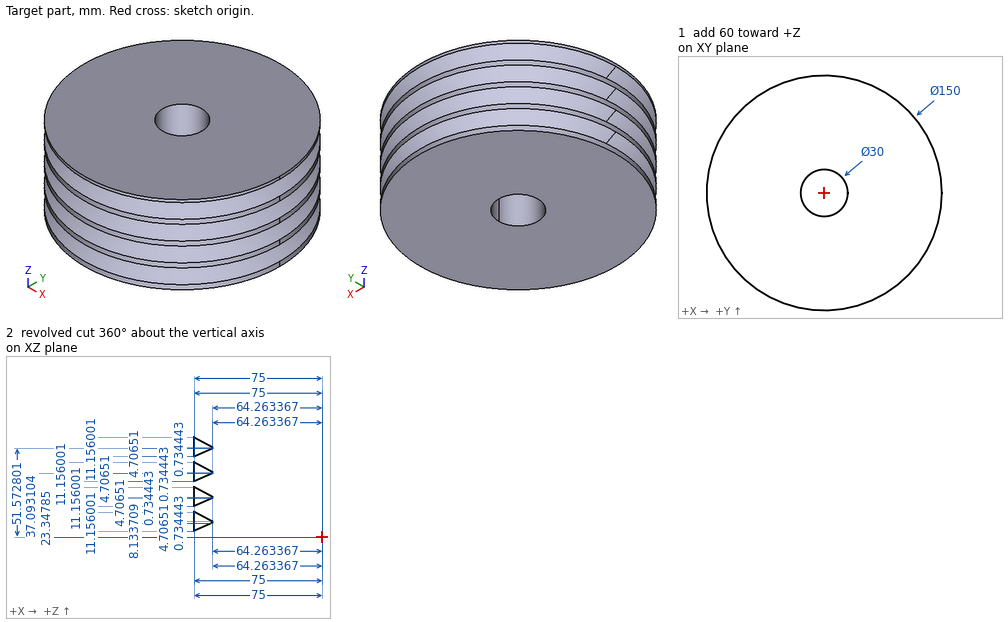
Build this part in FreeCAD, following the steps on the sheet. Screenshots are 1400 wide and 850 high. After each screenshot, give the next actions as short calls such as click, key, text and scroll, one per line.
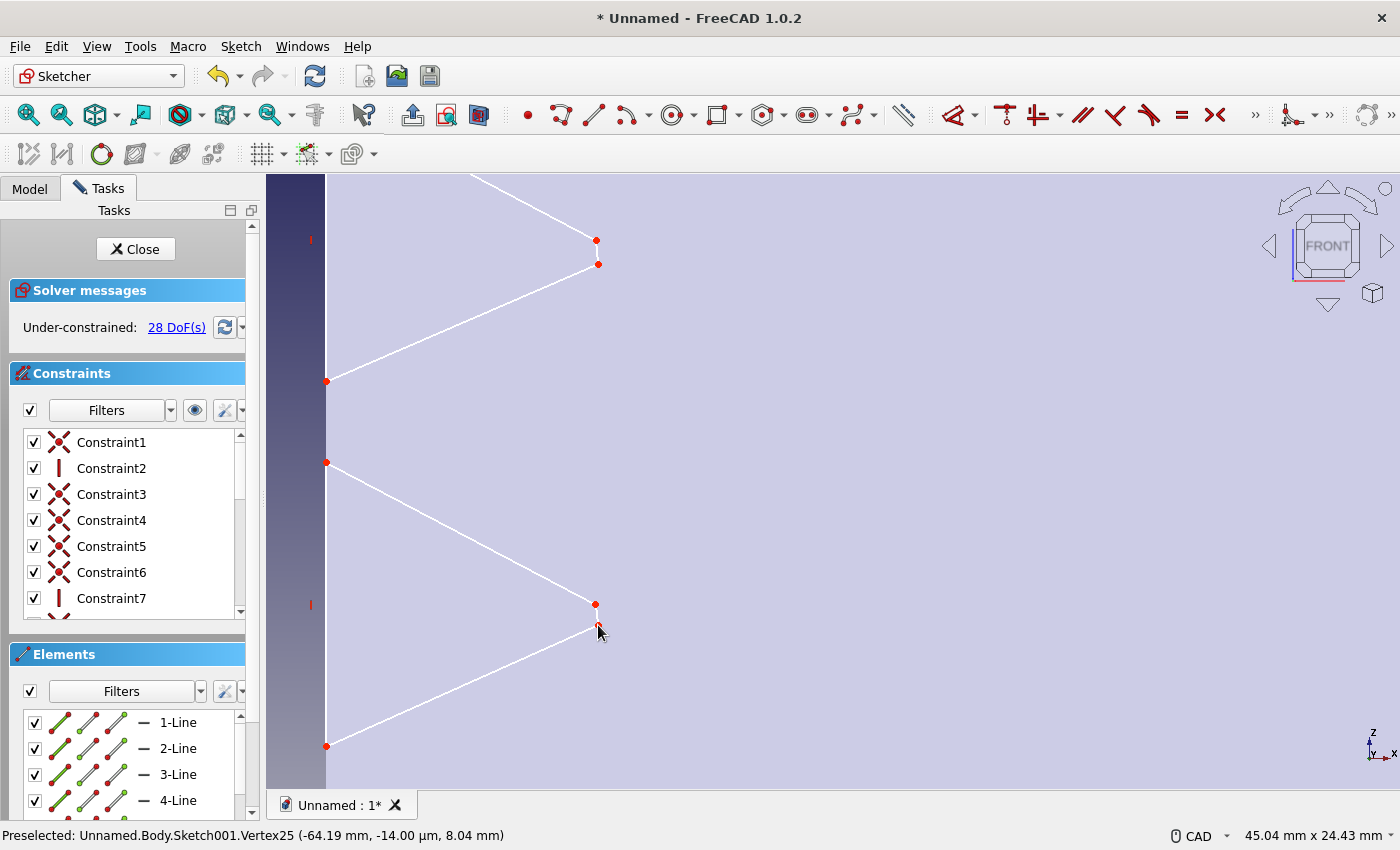
scroll(599, 607, down, 7)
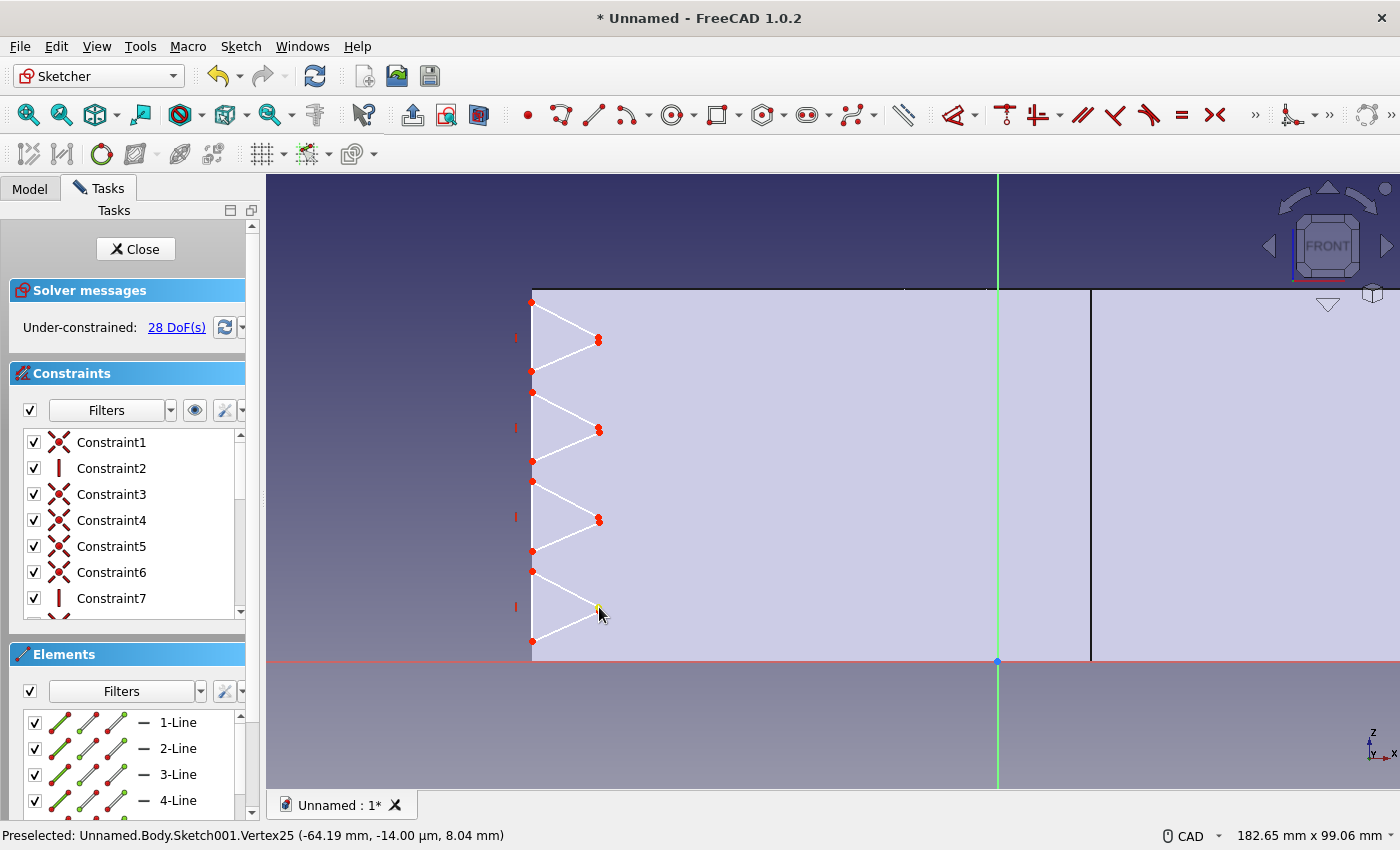
scroll(599, 340, up, 9)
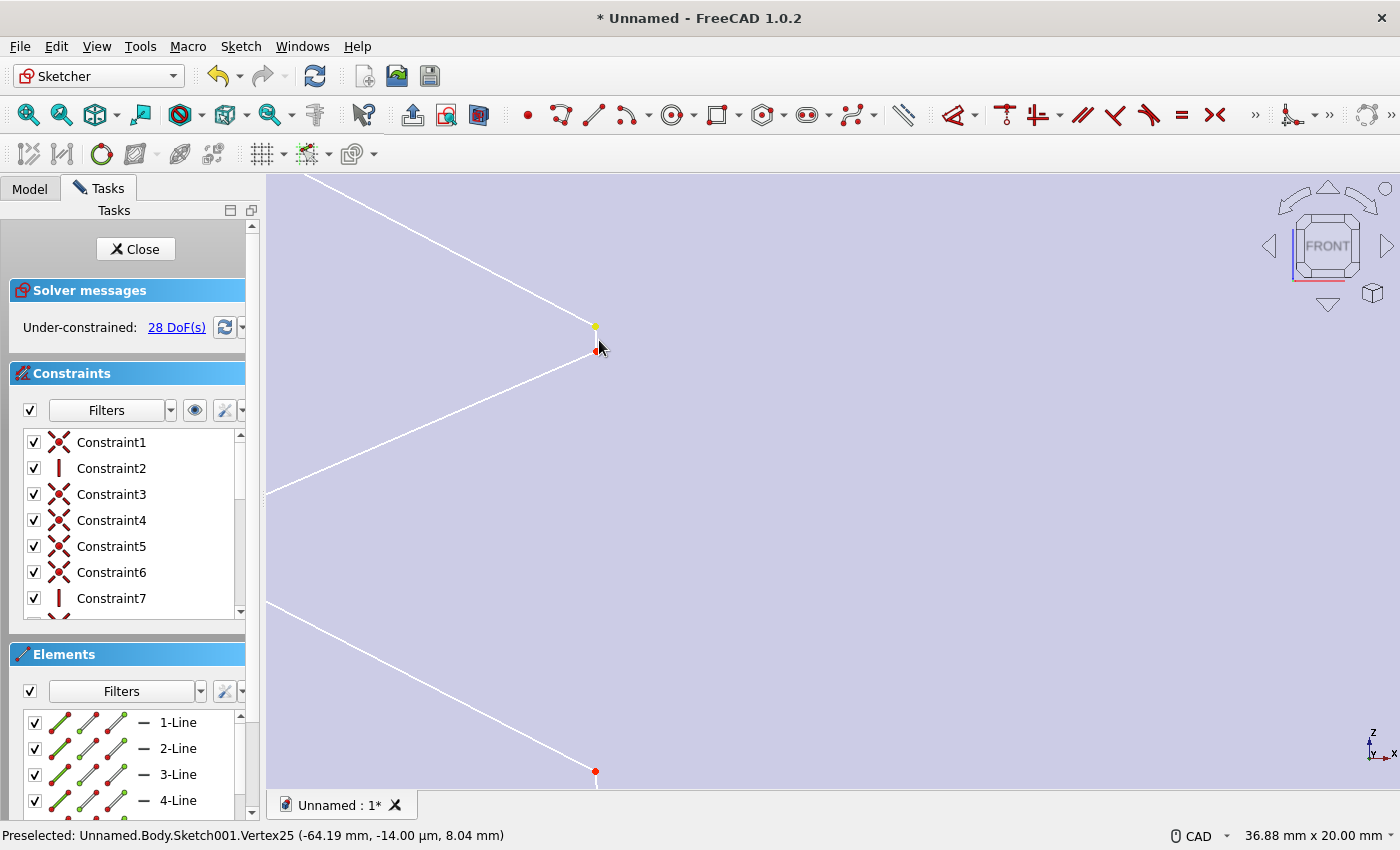
click(595, 339)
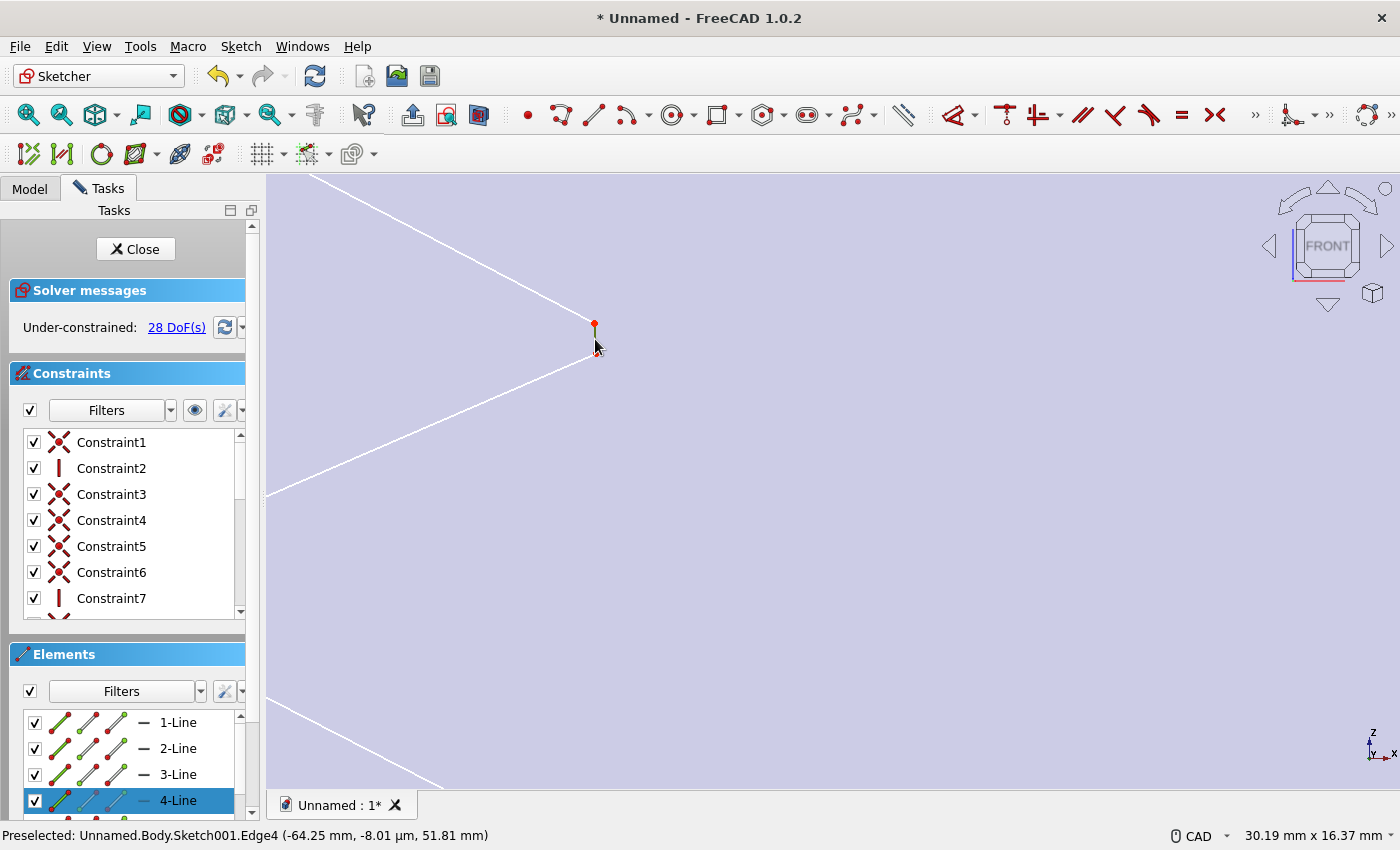
key(v)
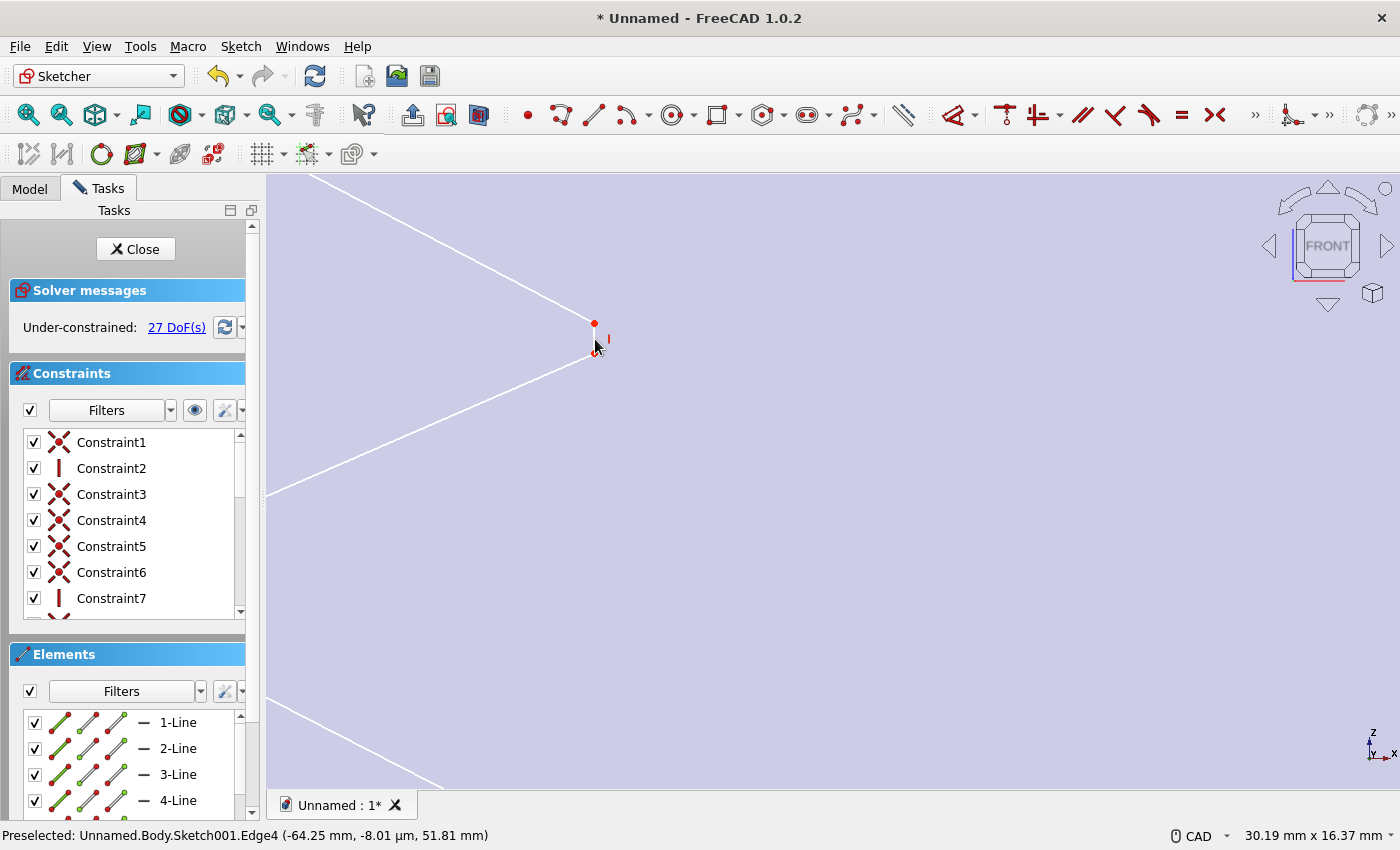
scroll(599, 340, down, 9)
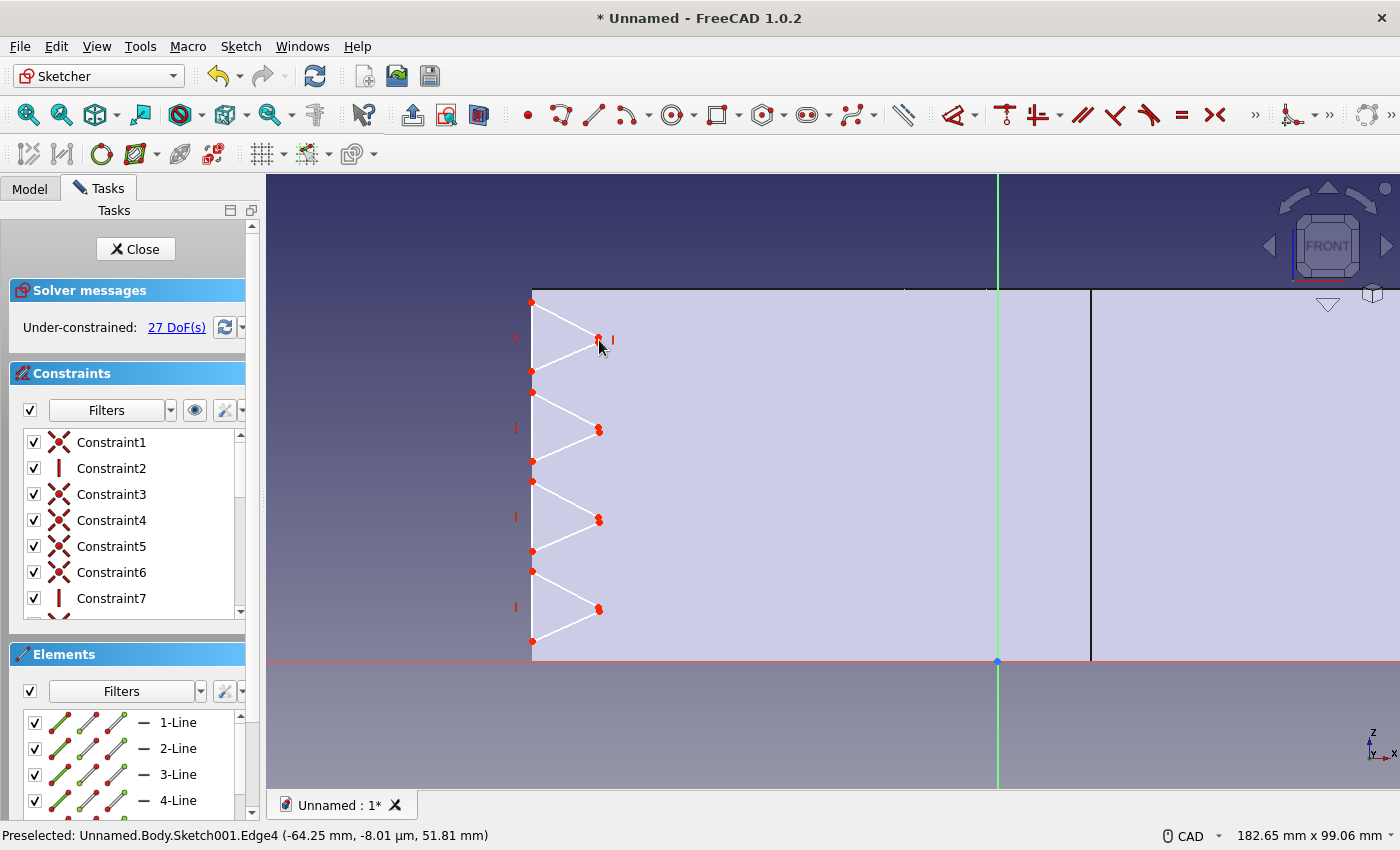
scroll(599, 429, up, 11)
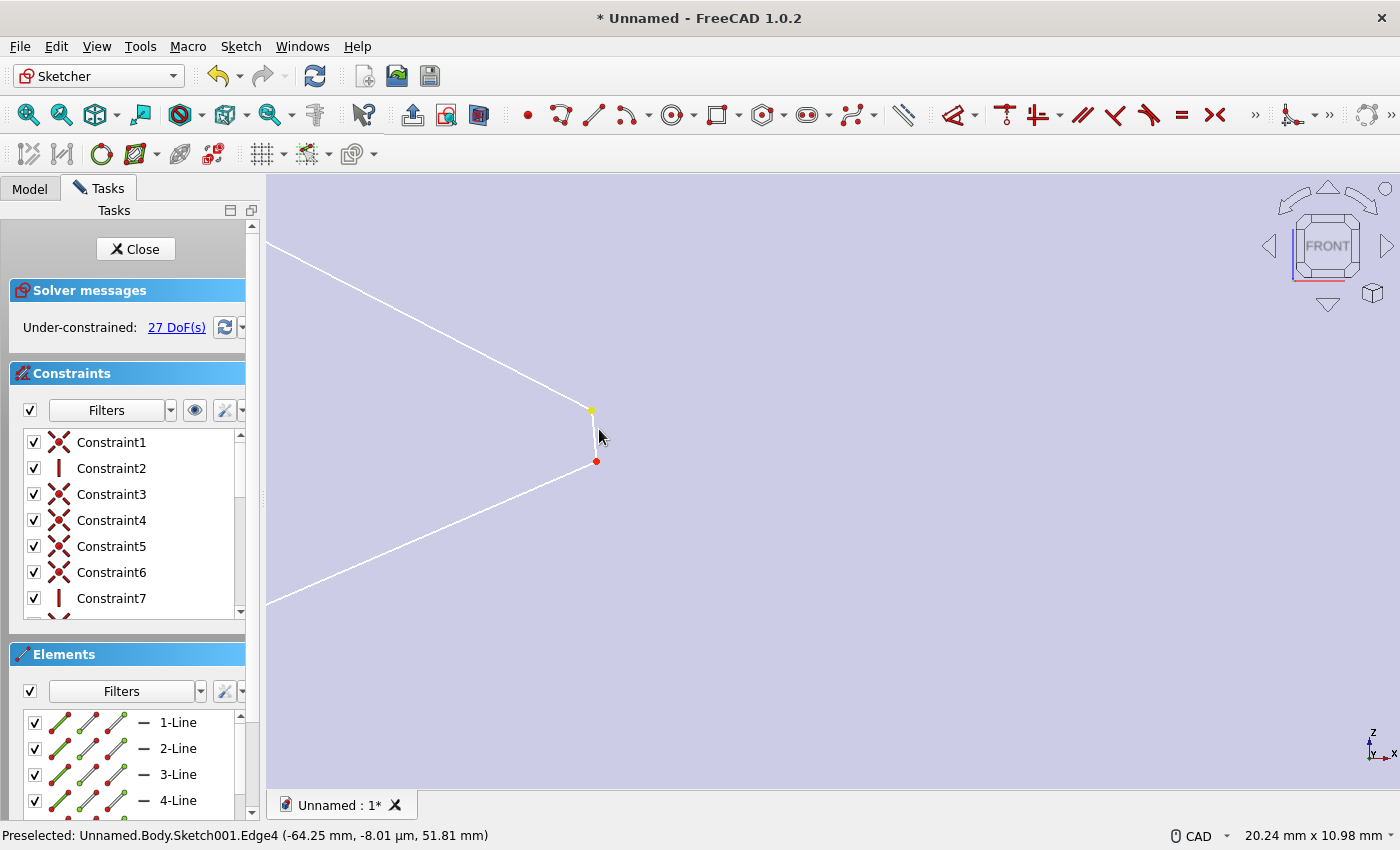
click(593, 426)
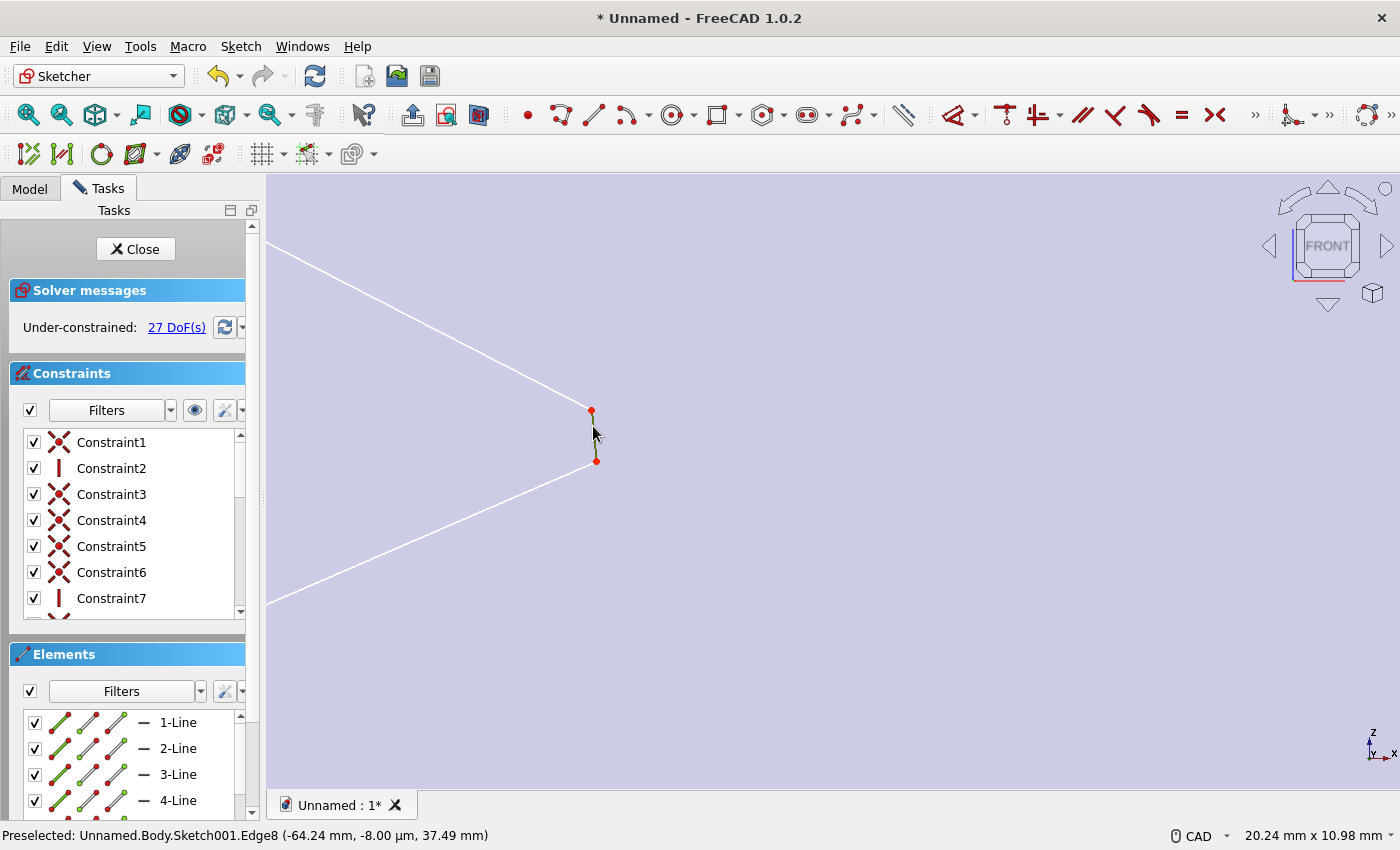
click(1060, 116)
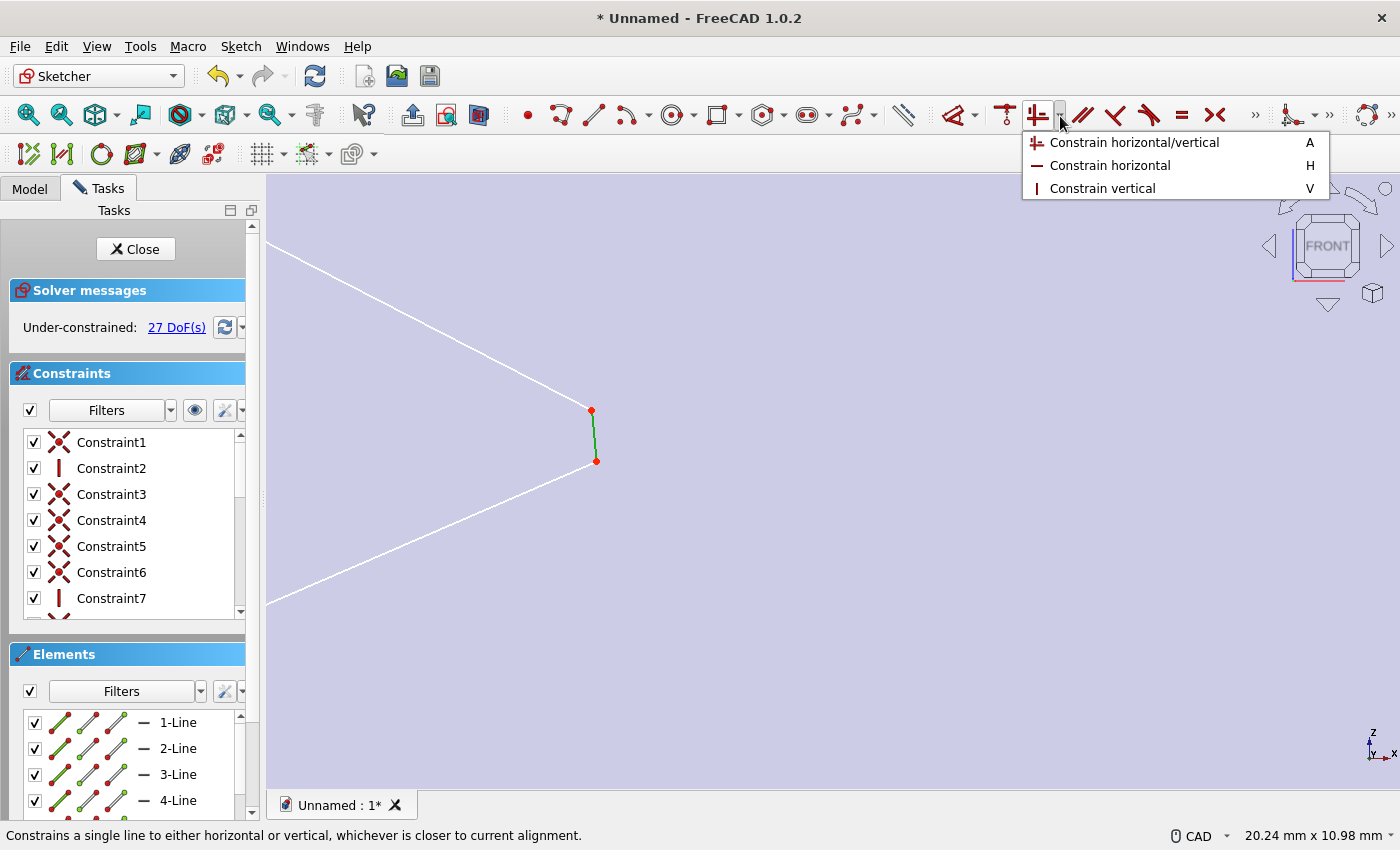
click(1176, 188)